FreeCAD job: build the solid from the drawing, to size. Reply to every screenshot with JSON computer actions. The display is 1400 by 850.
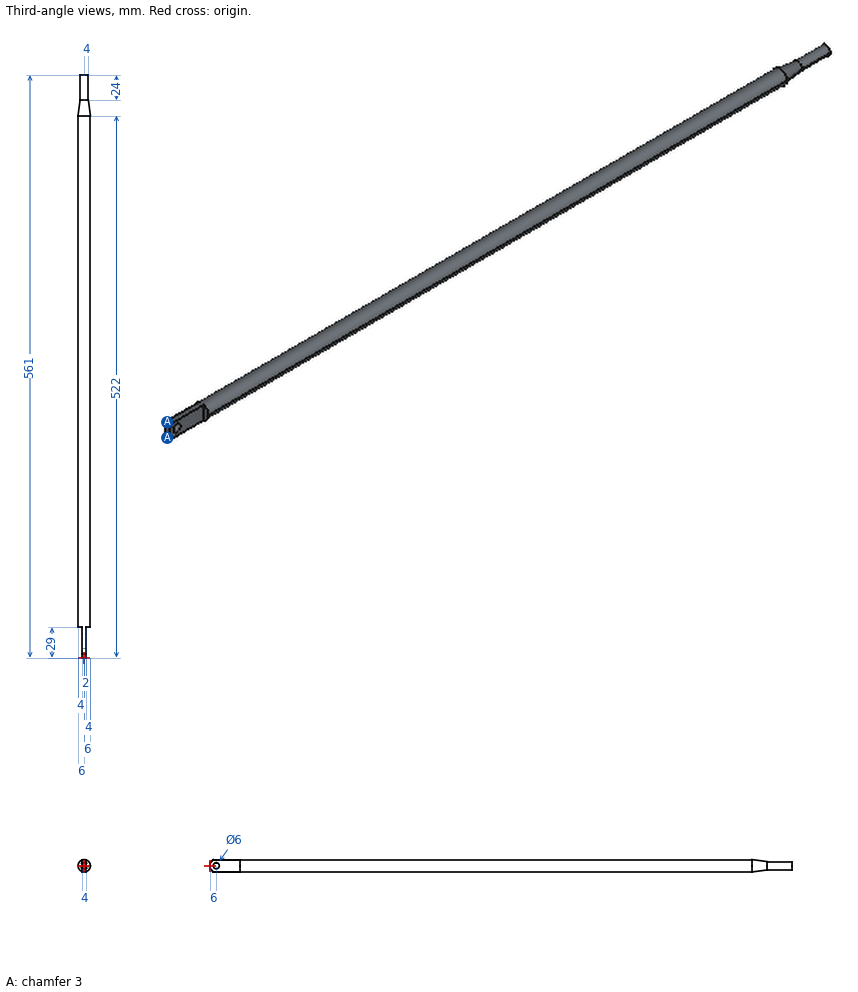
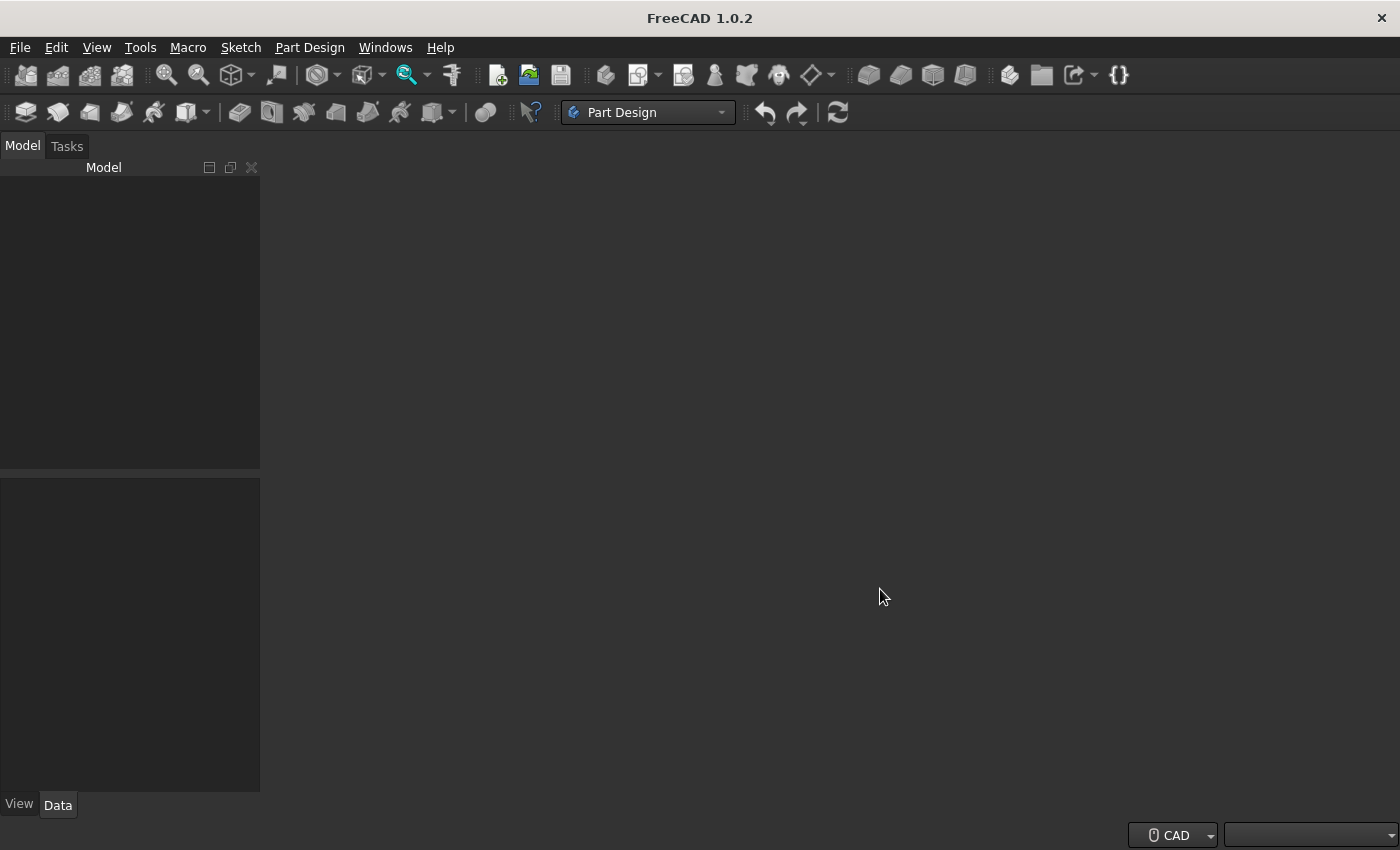
{"action": "left_click", "coordinate": [498, 76]}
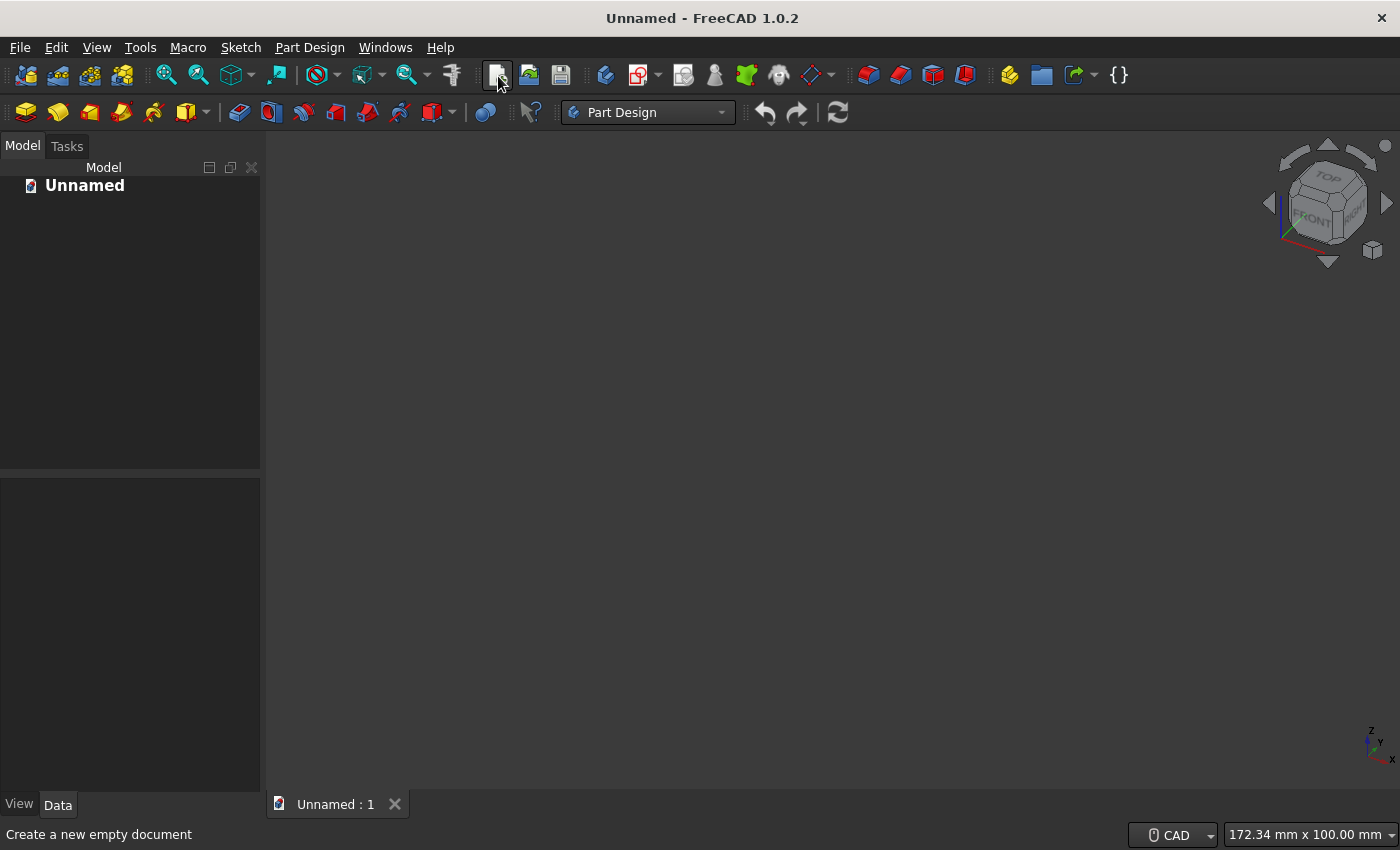
{"action": "left_click", "coordinate": [638, 76]}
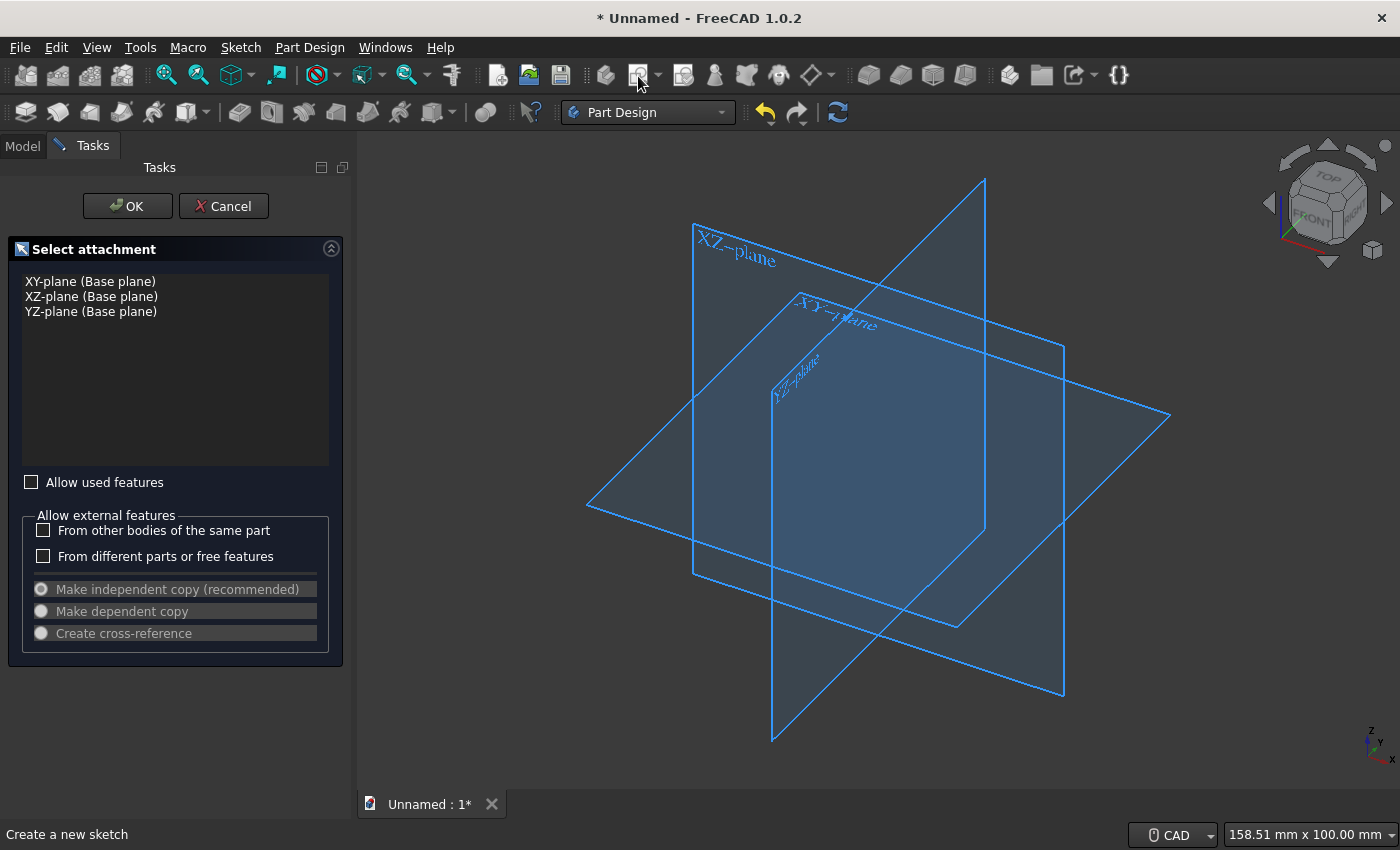
{"action": "left_click", "coordinate": [82, 282]}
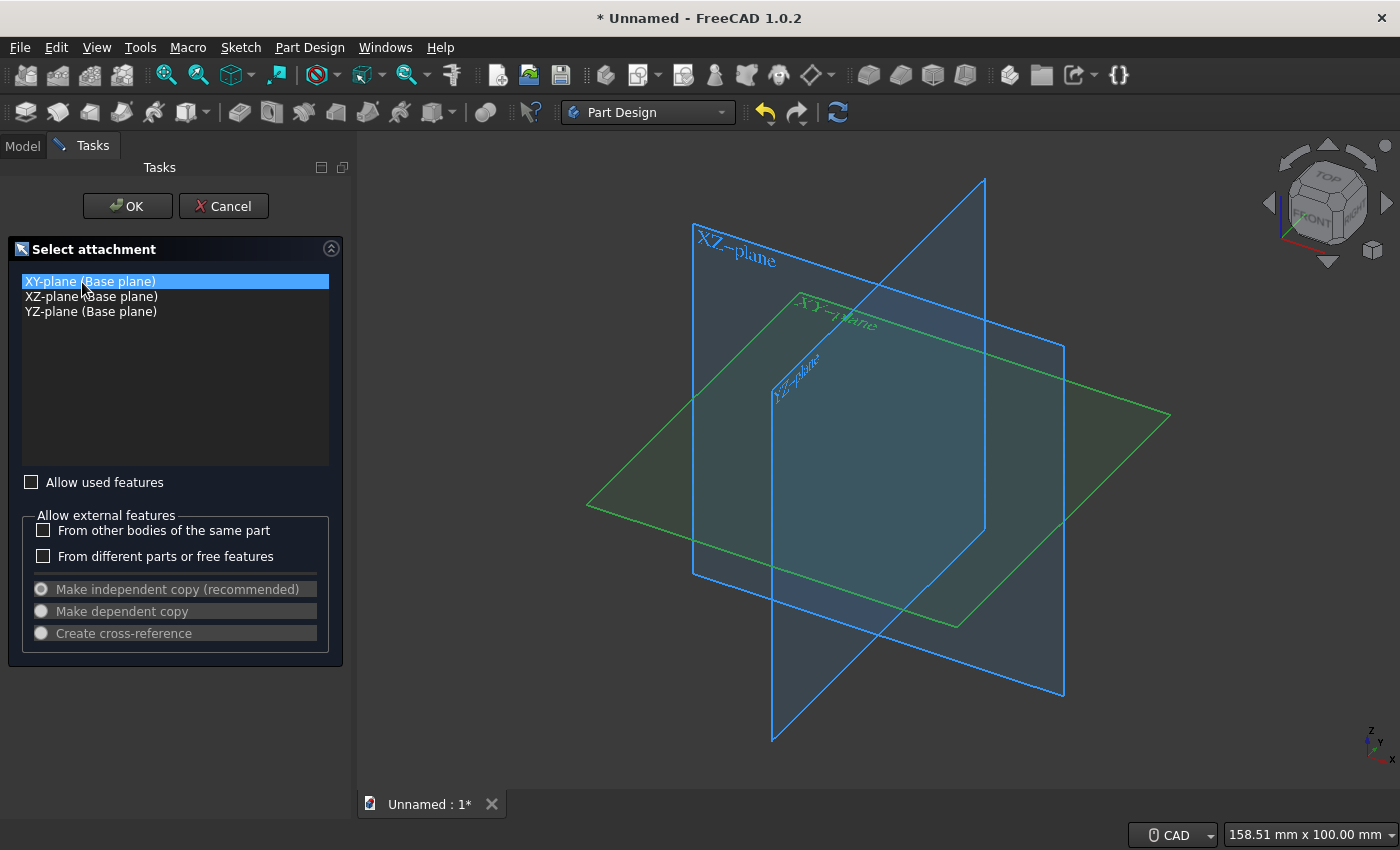
{"action": "left_click", "coordinate": [128, 206]}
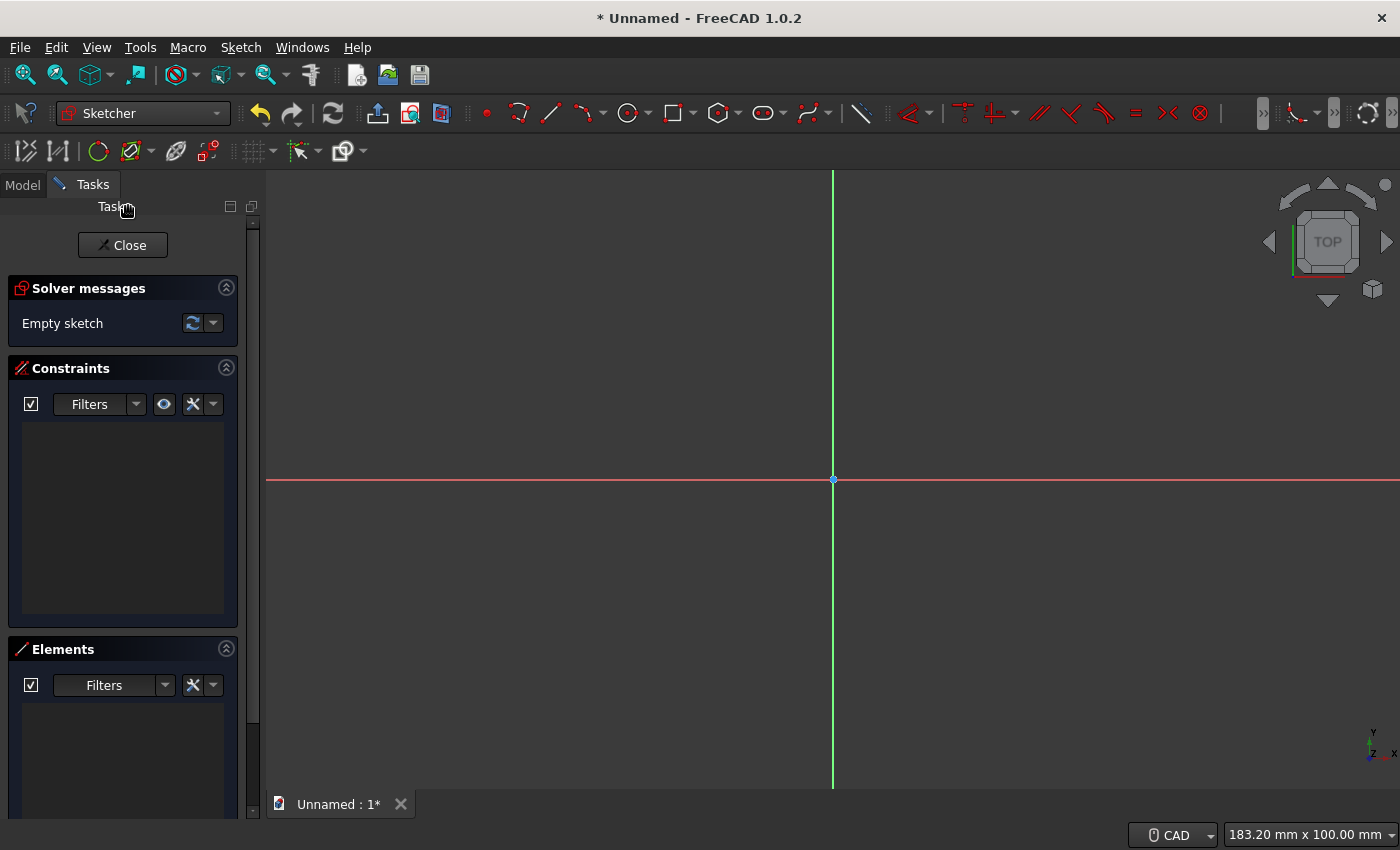
{"action": "scroll", "coordinate": [754, 696], "scroll_direction": "down", "scroll_amount": 11}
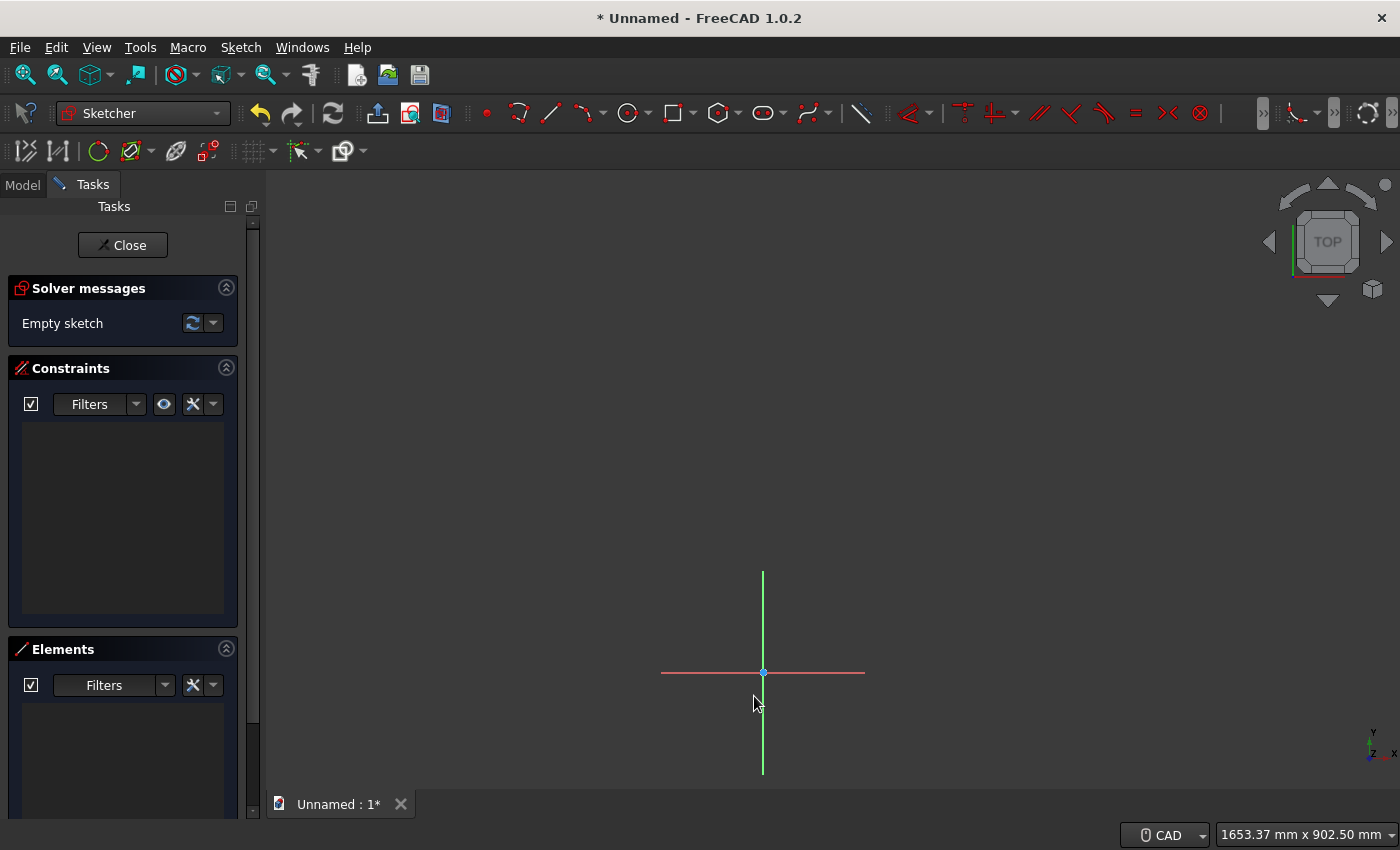
{"action": "left_click", "coordinate": [520, 114]}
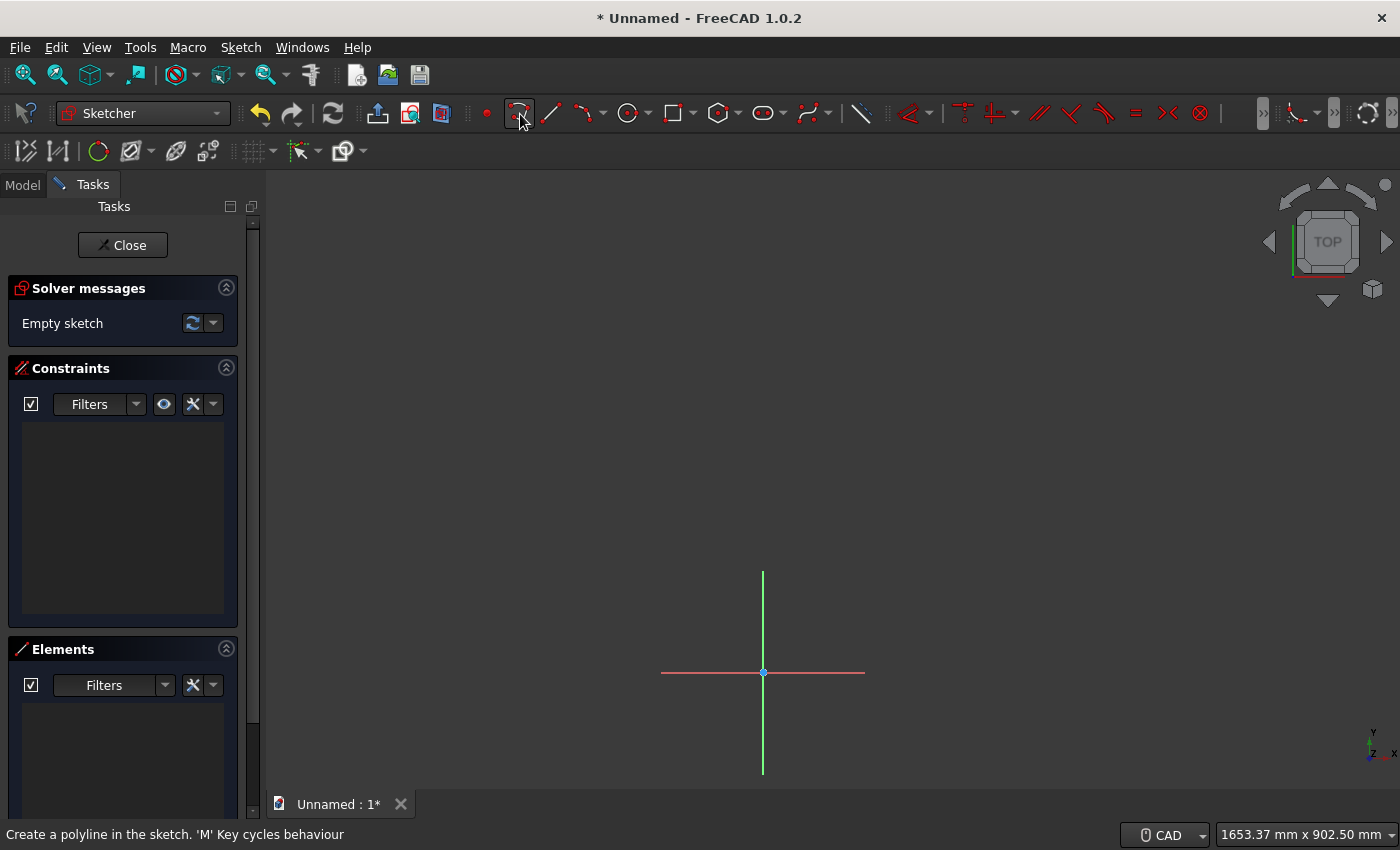
{"action": "left_click", "coordinate": [763, 673]}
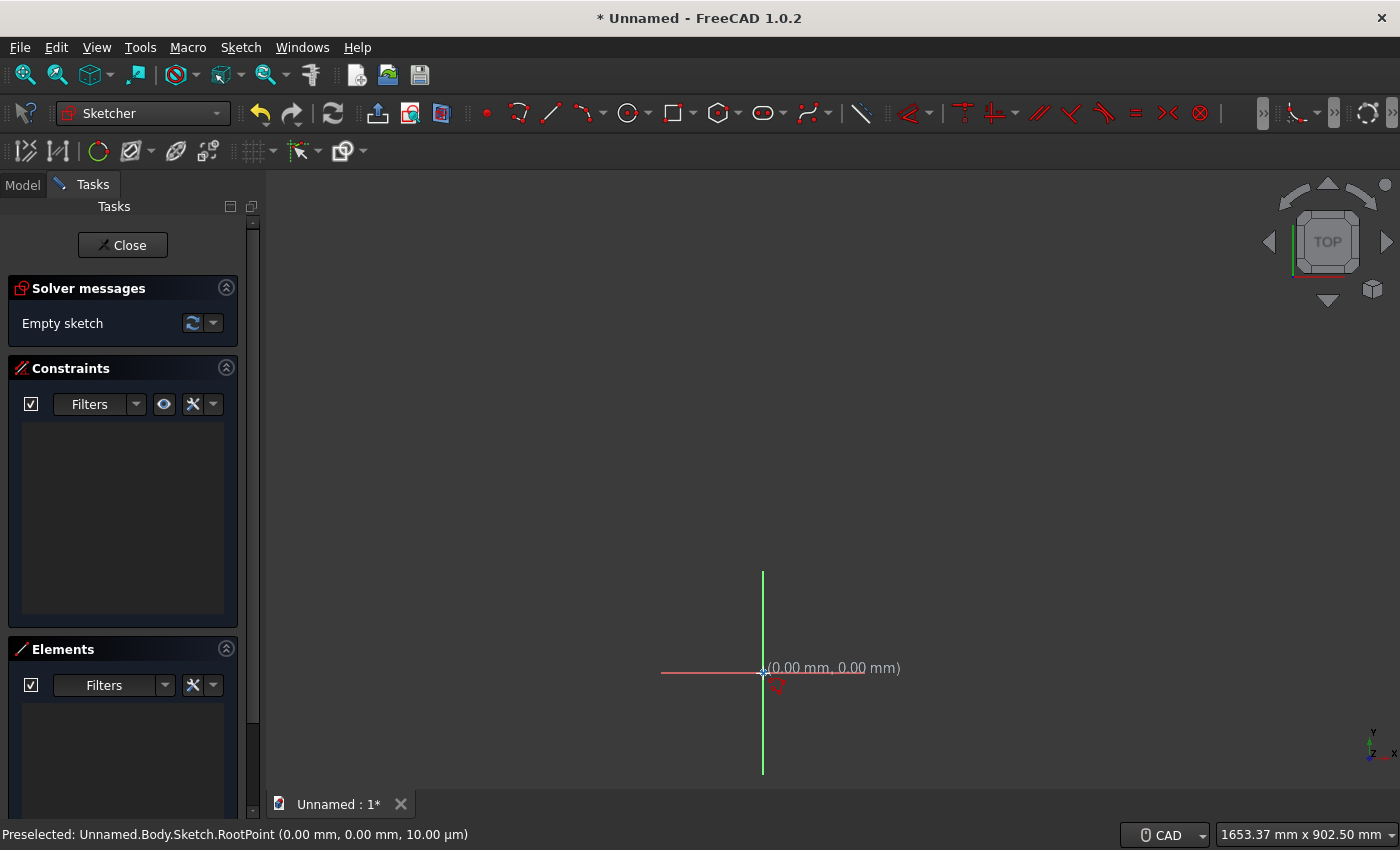
{"action": "scroll", "coordinate": [767, 673], "scroll_direction": "up", "scroll_amount": 7}